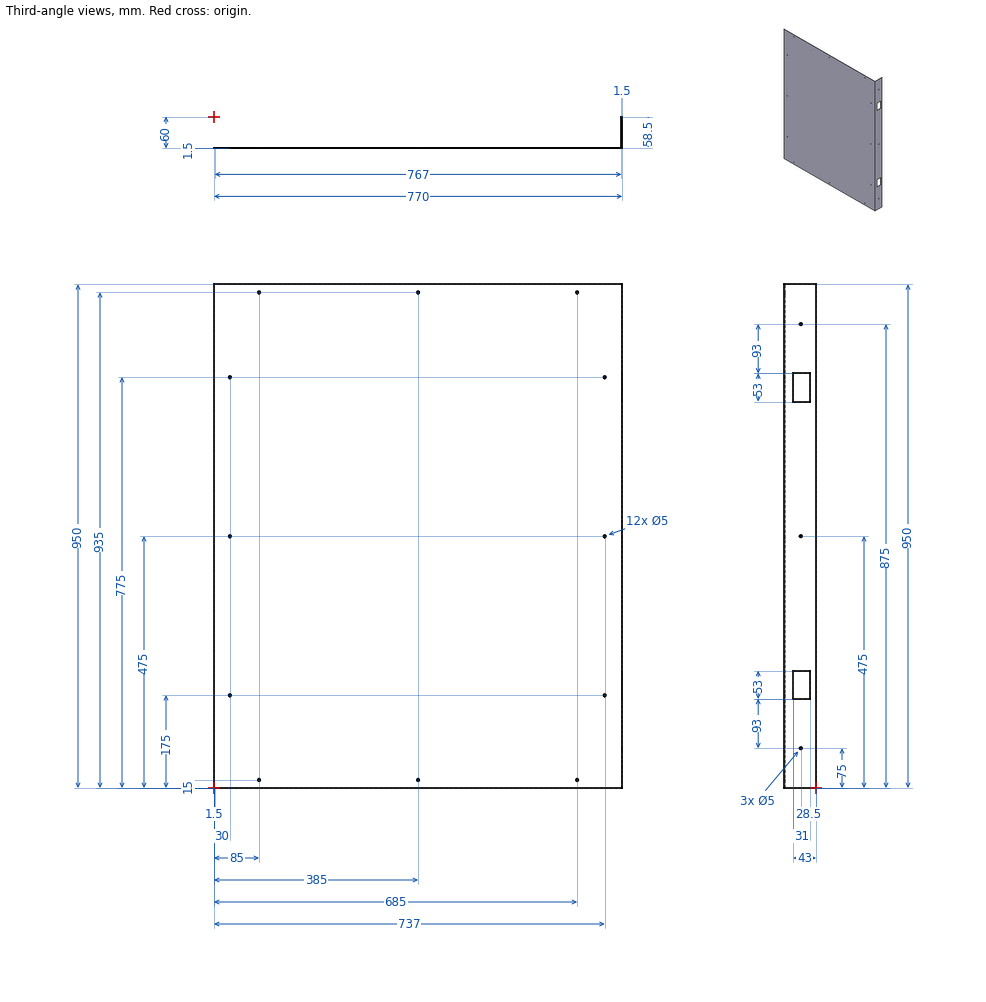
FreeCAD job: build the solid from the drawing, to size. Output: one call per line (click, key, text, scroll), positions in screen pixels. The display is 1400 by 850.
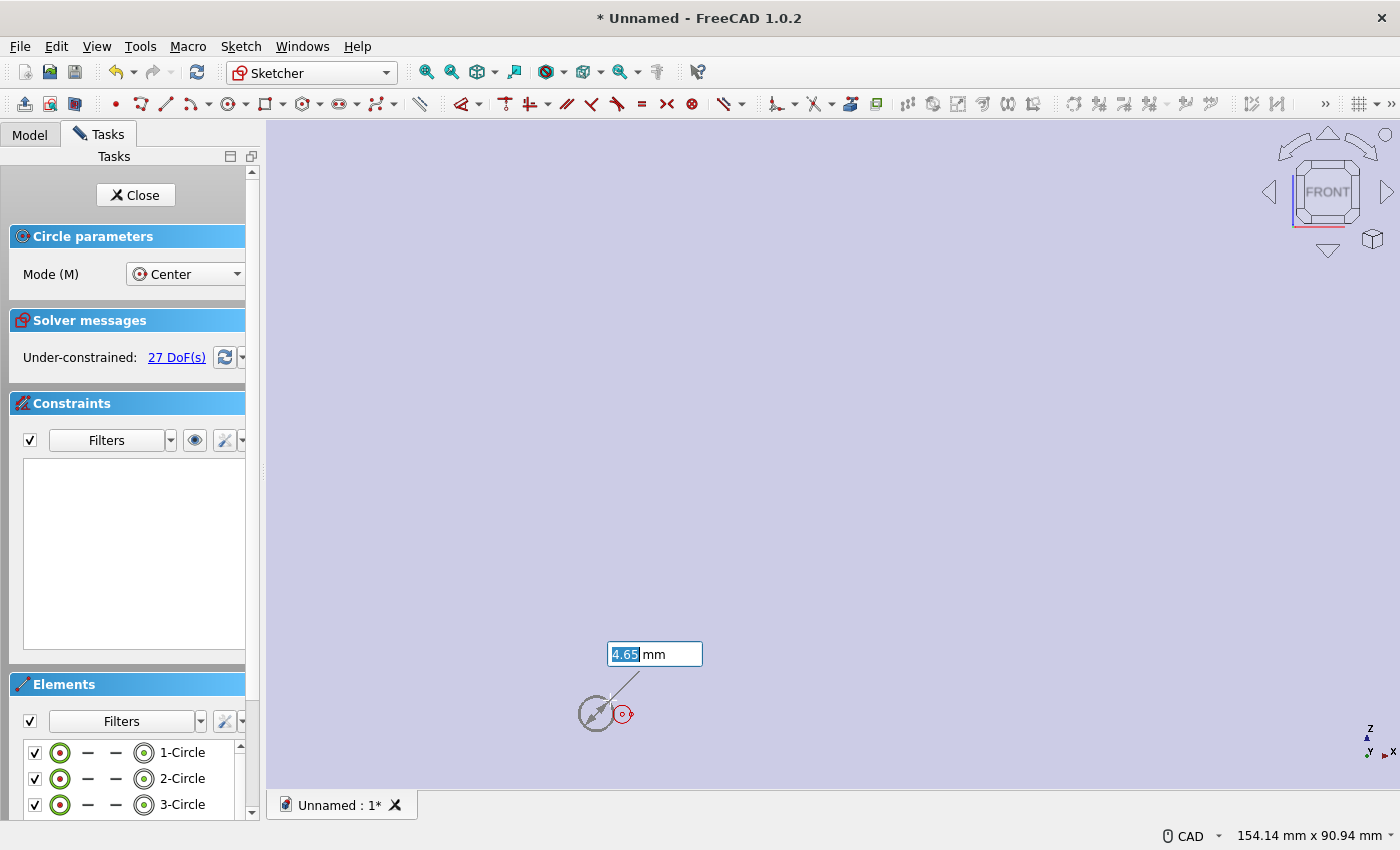
click(610, 694)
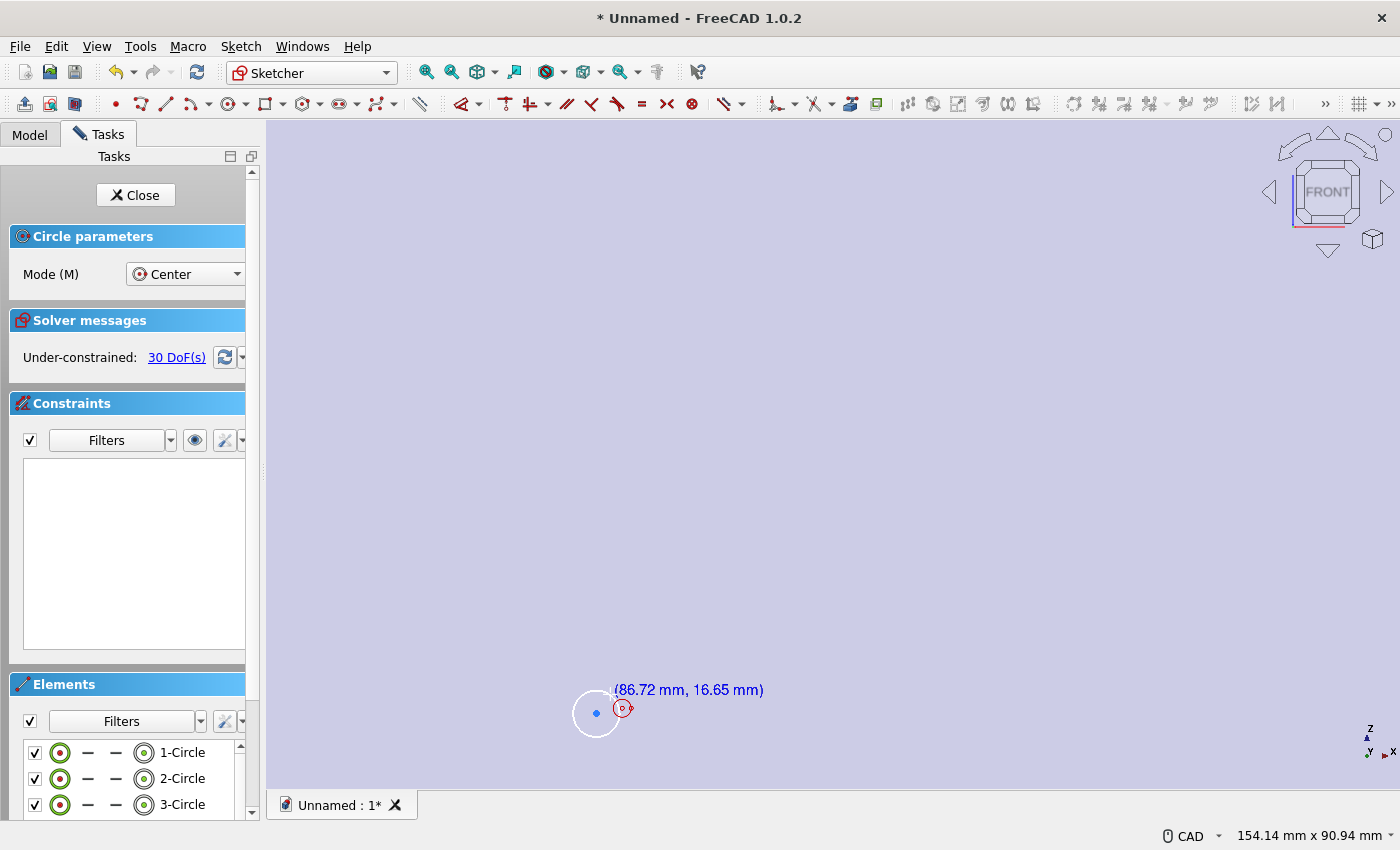
scroll(640, 654, down, 14)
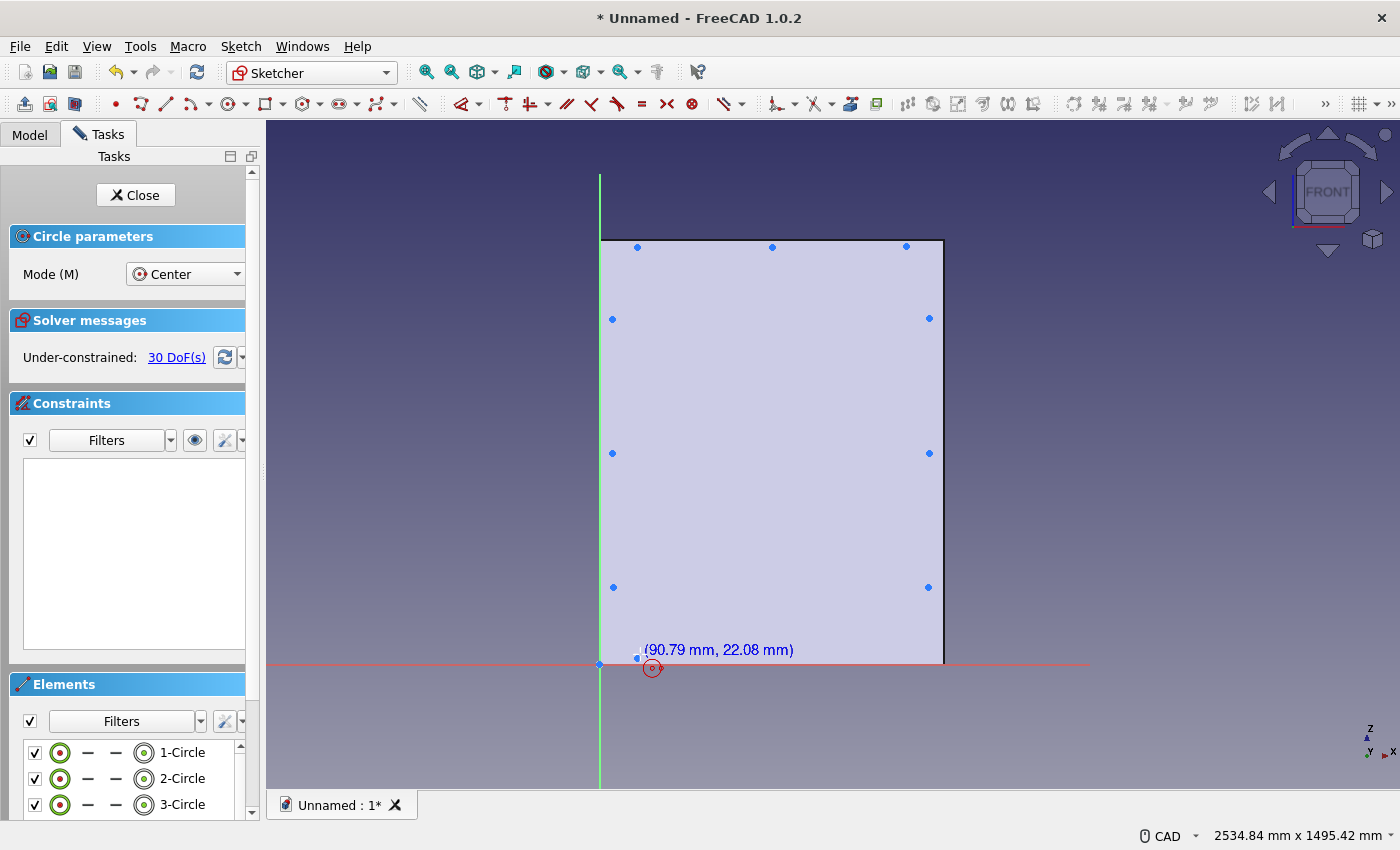
scroll(906, 658, up, 16)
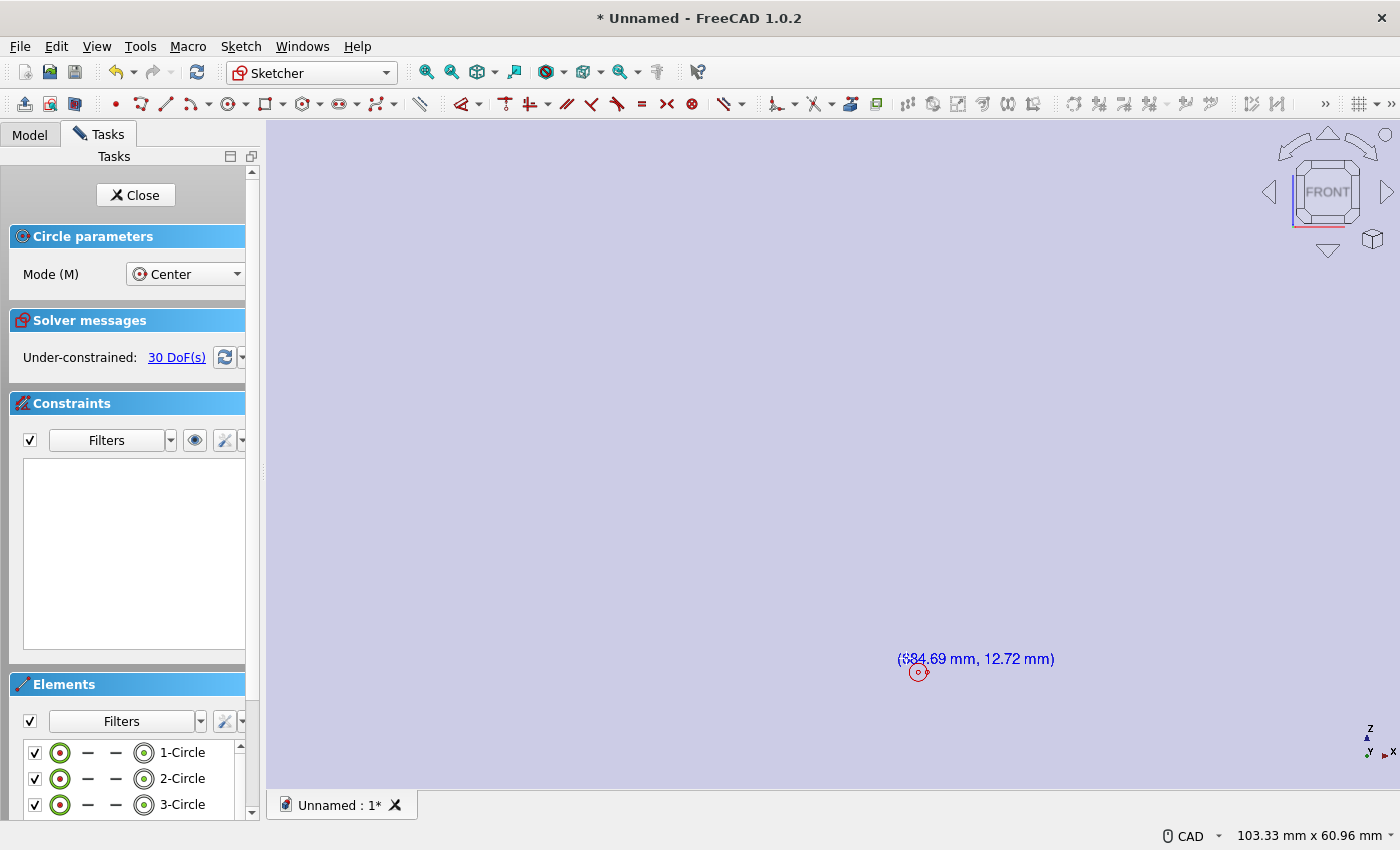
scroll(939, 706, down, 15)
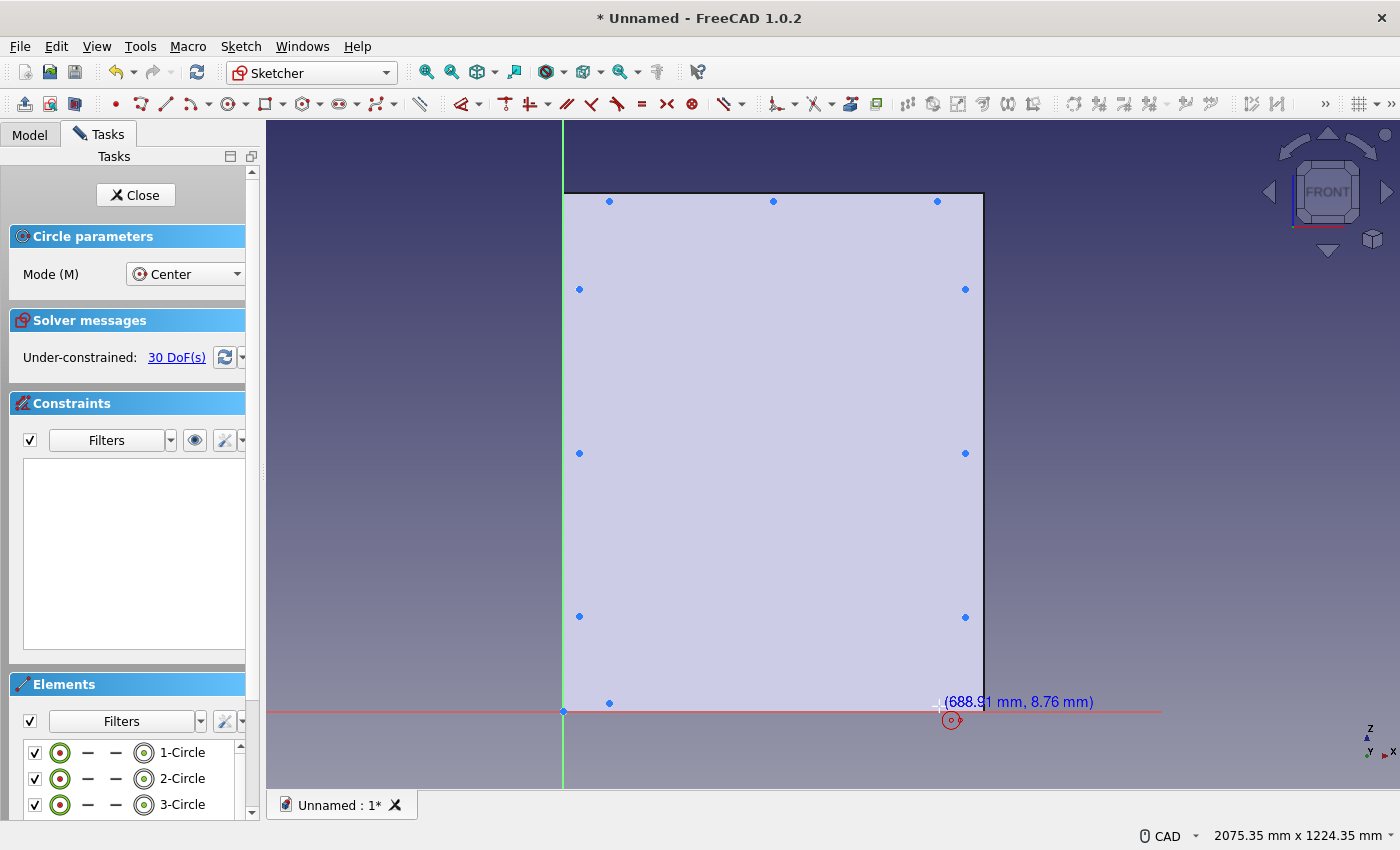
scroll(937, 703, up, 4)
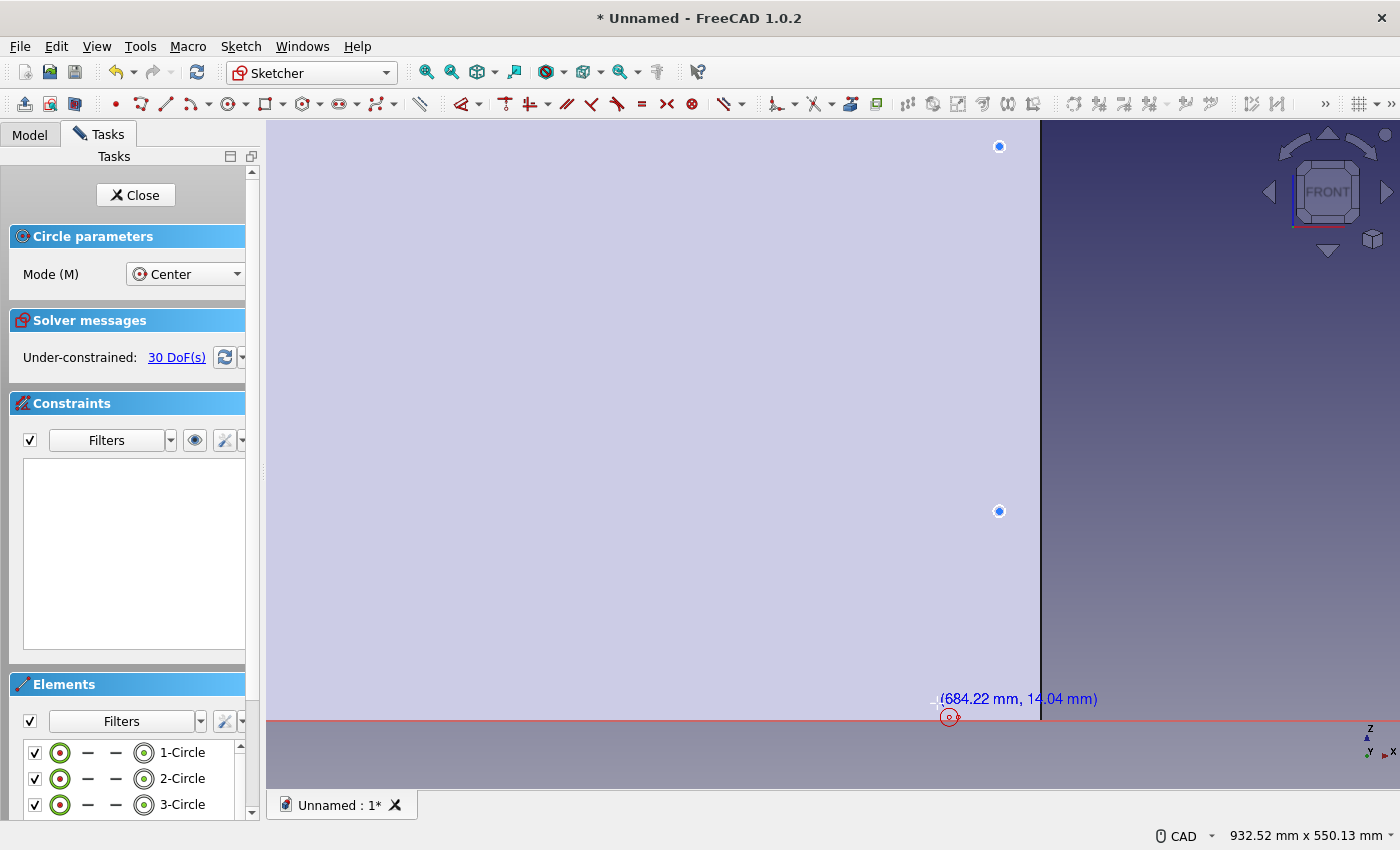
click(937, 703)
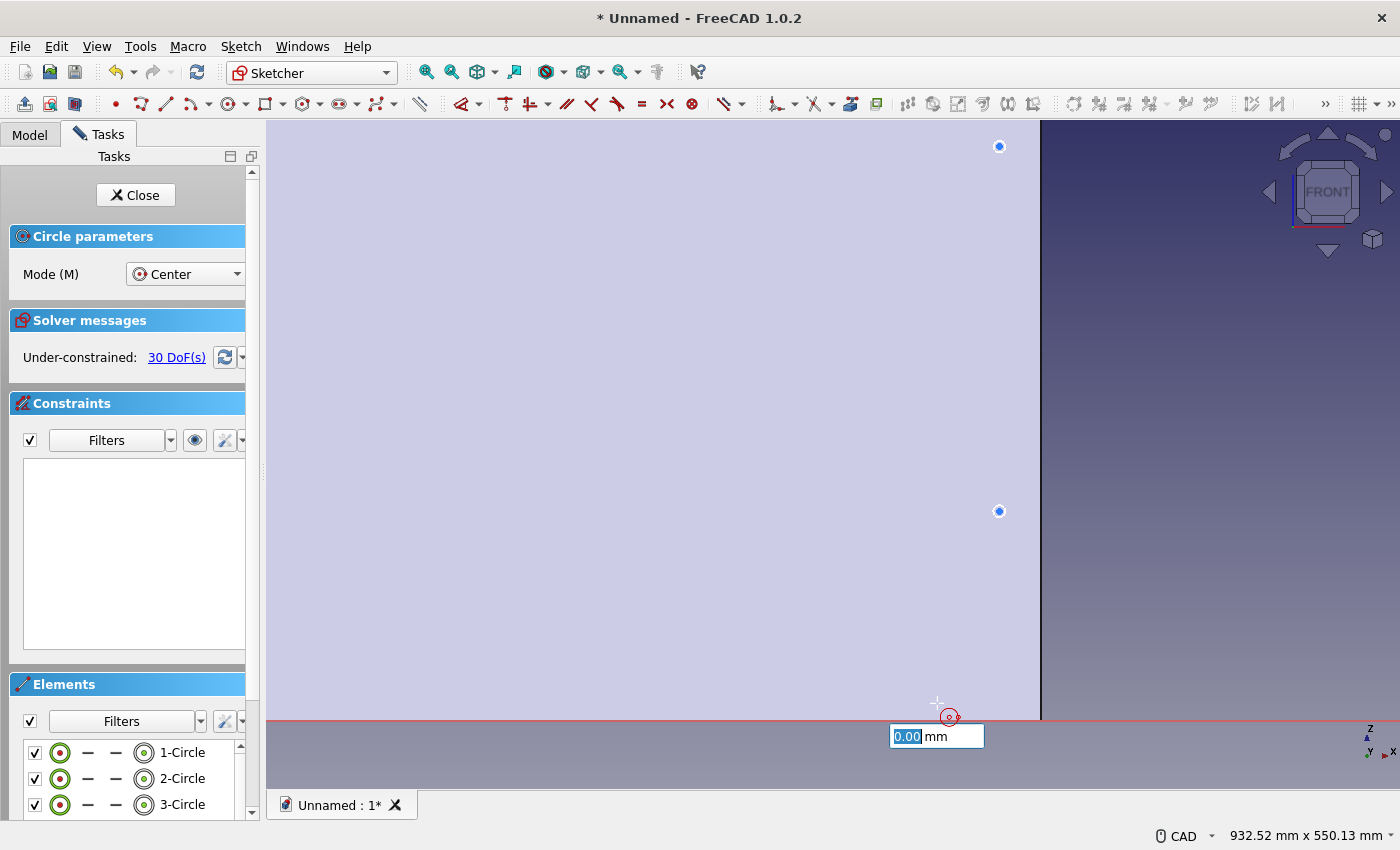
scroll(939, 701, up, 9)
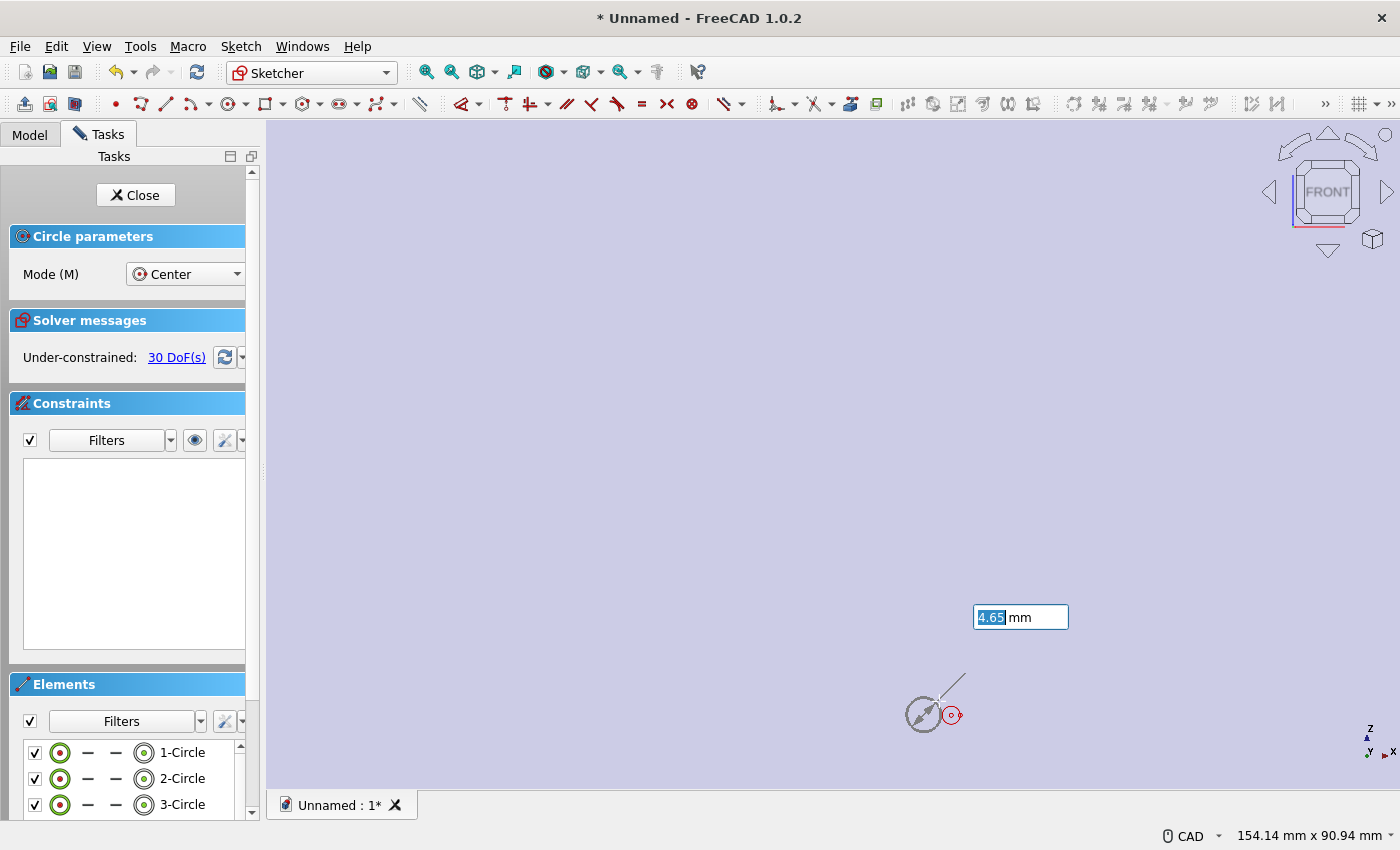
click(938, 696)